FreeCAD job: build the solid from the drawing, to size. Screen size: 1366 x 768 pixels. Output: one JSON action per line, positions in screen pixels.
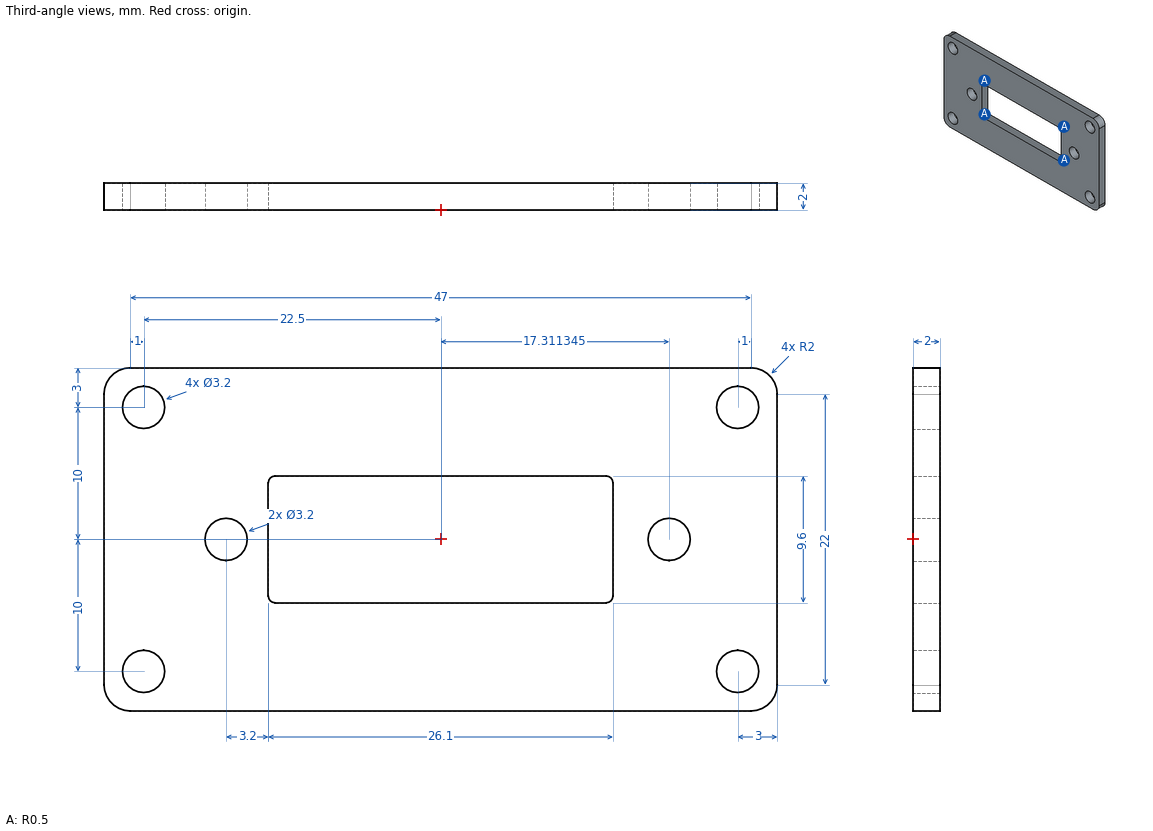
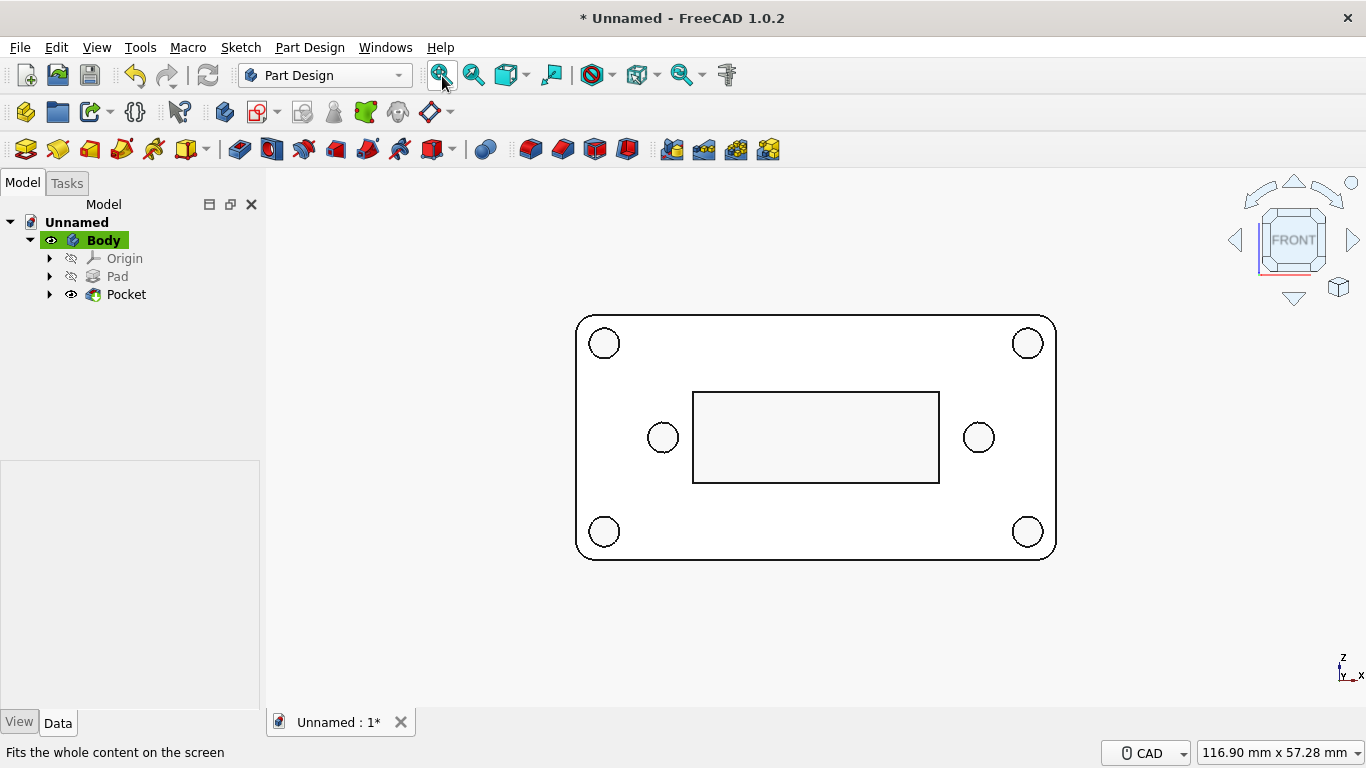
{"action": "key", "text": "3"}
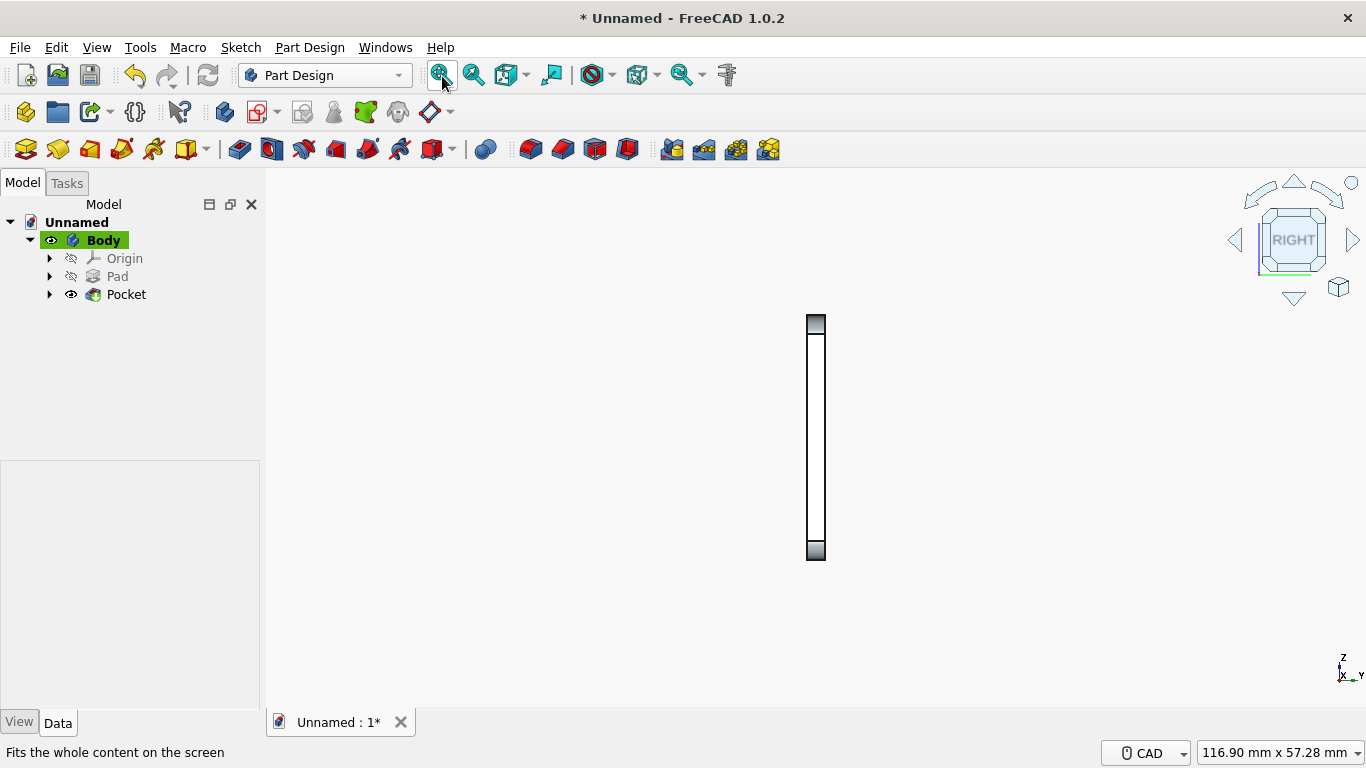
{"action": "scroll", "coordinate": [816, 391], "scroll_direction": "up", "scroll_amount": 4}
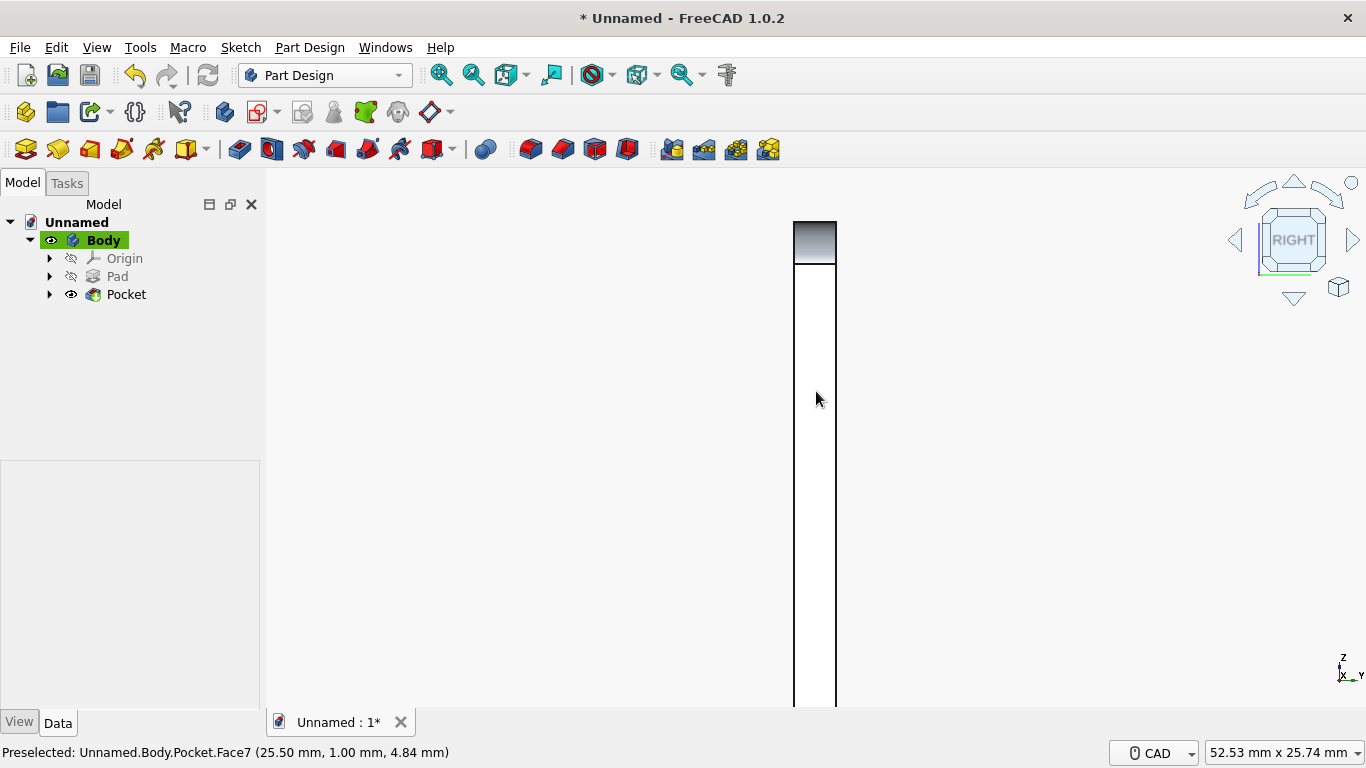
{"action": "left_click", "coordinate": [442, 76]}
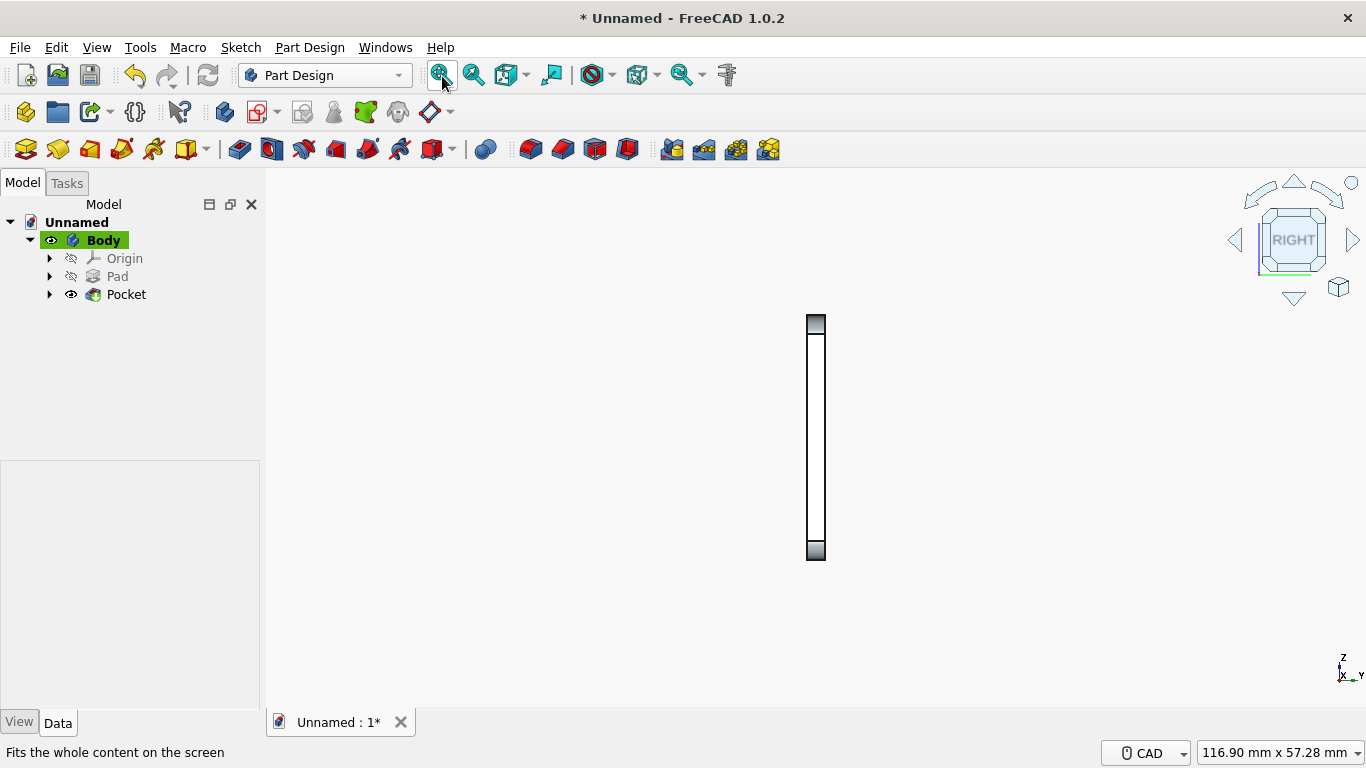
{"action": "key", "text": "5"}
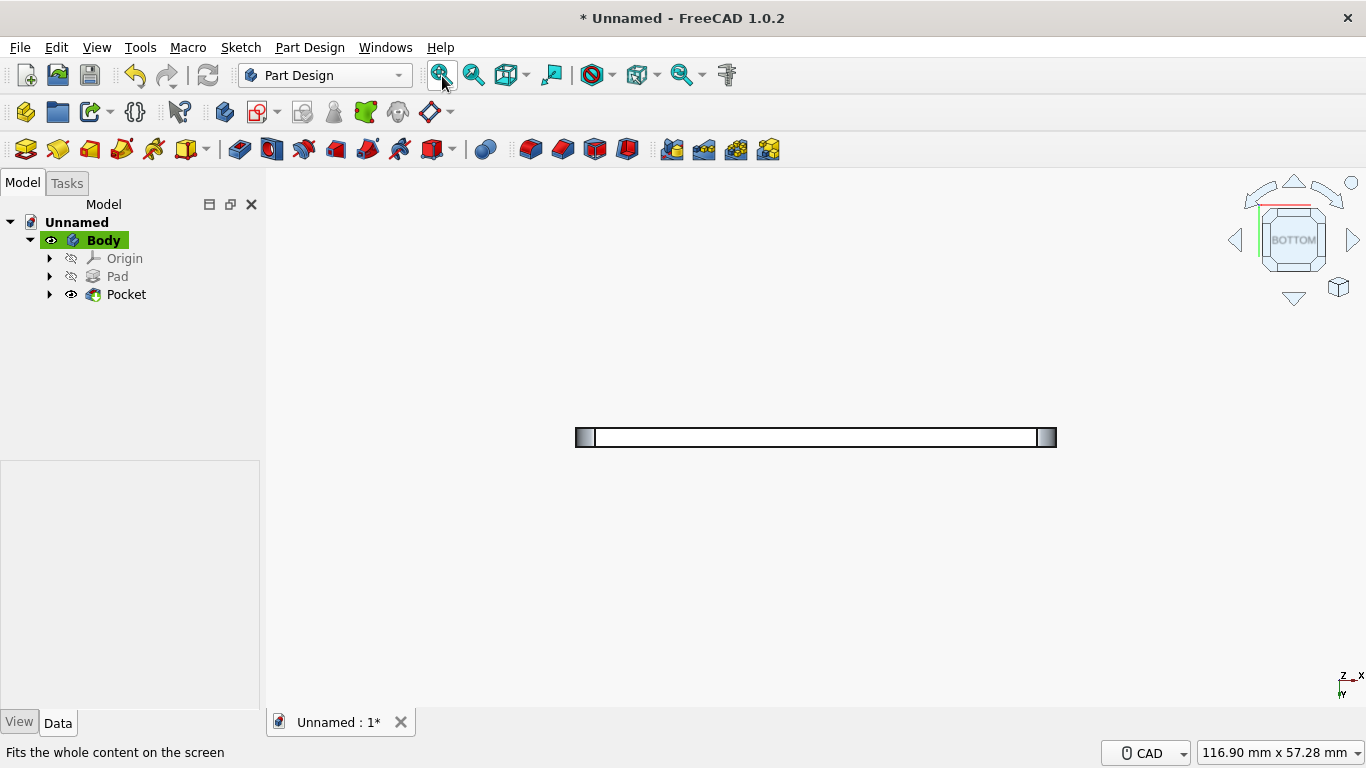
{"action": "left_click", "coordinate": [442, 76]}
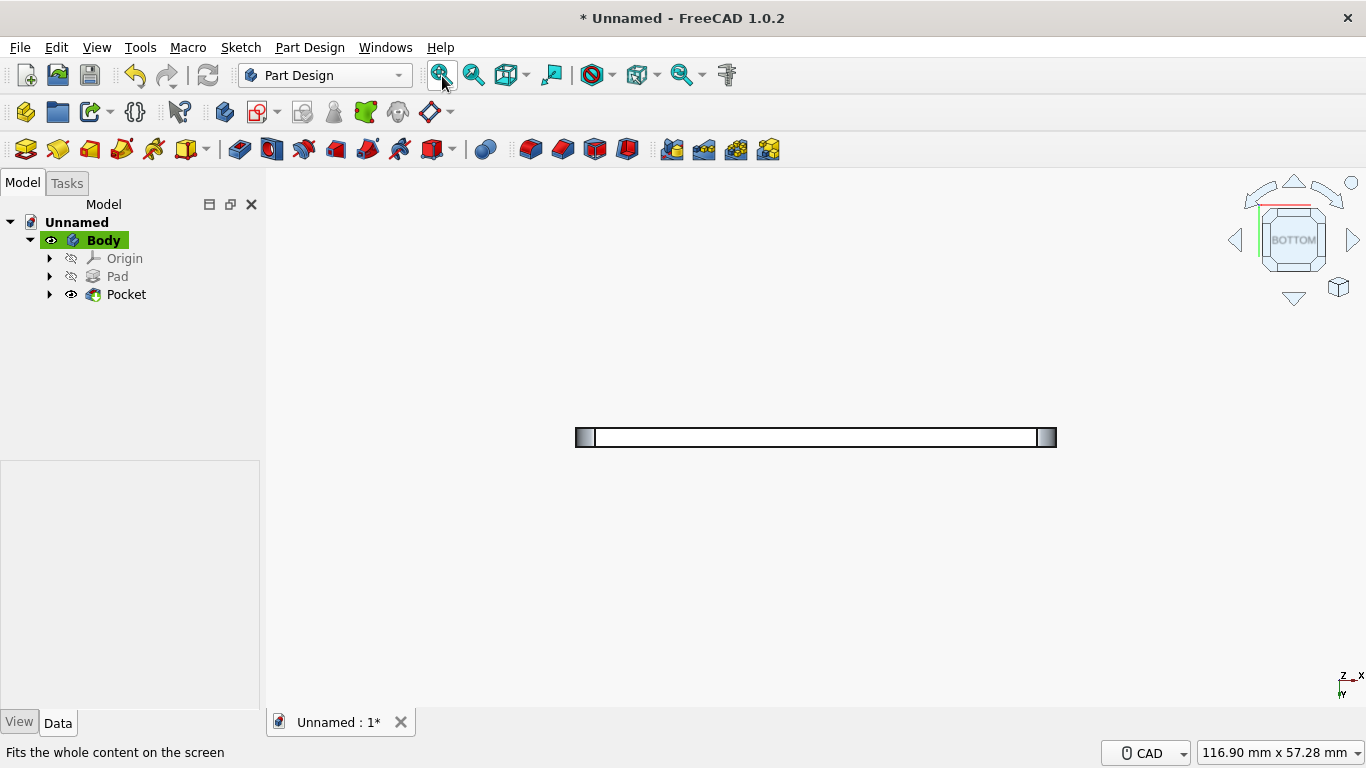
{"action": "scroll", "coordinate": [939, 436], "scroll_direction": "up", "scroll_amount": 4}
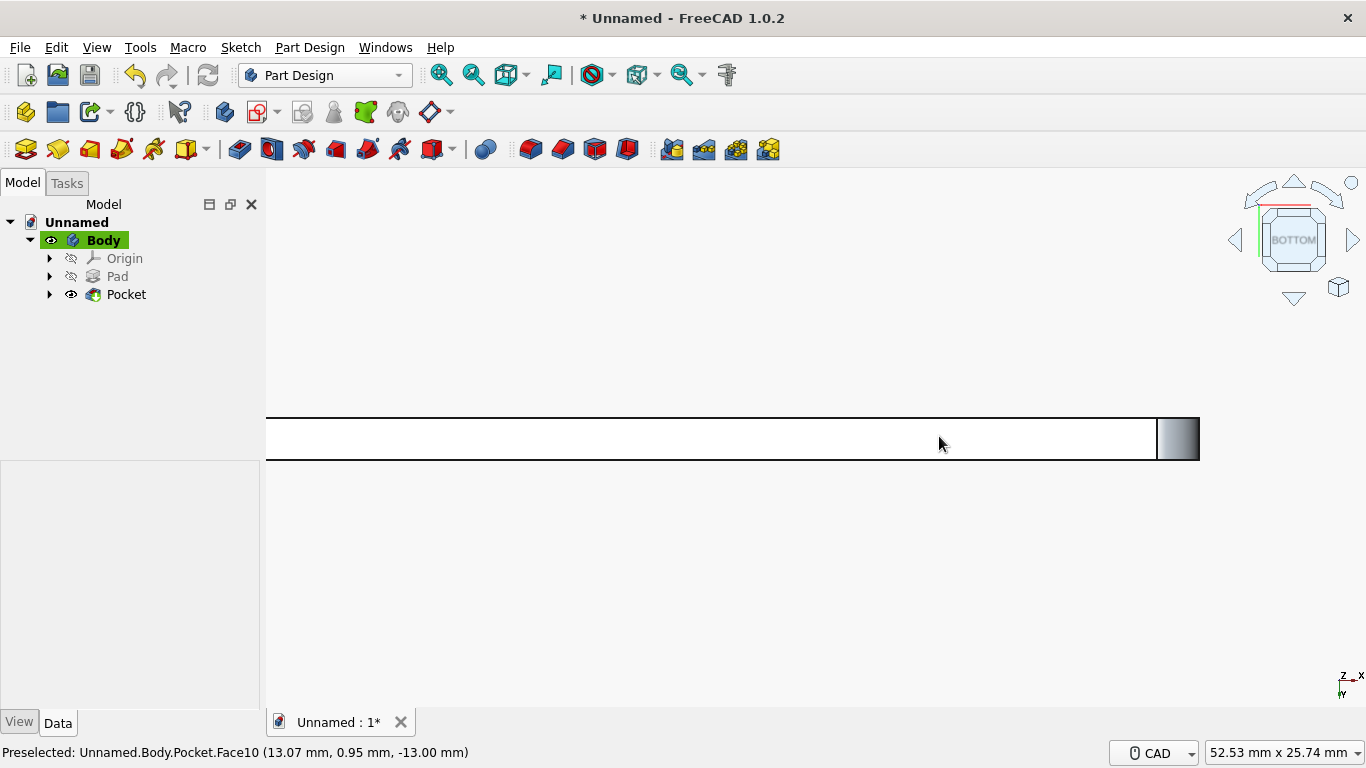
{"action": "left_click", "coordinate": [442, 76]}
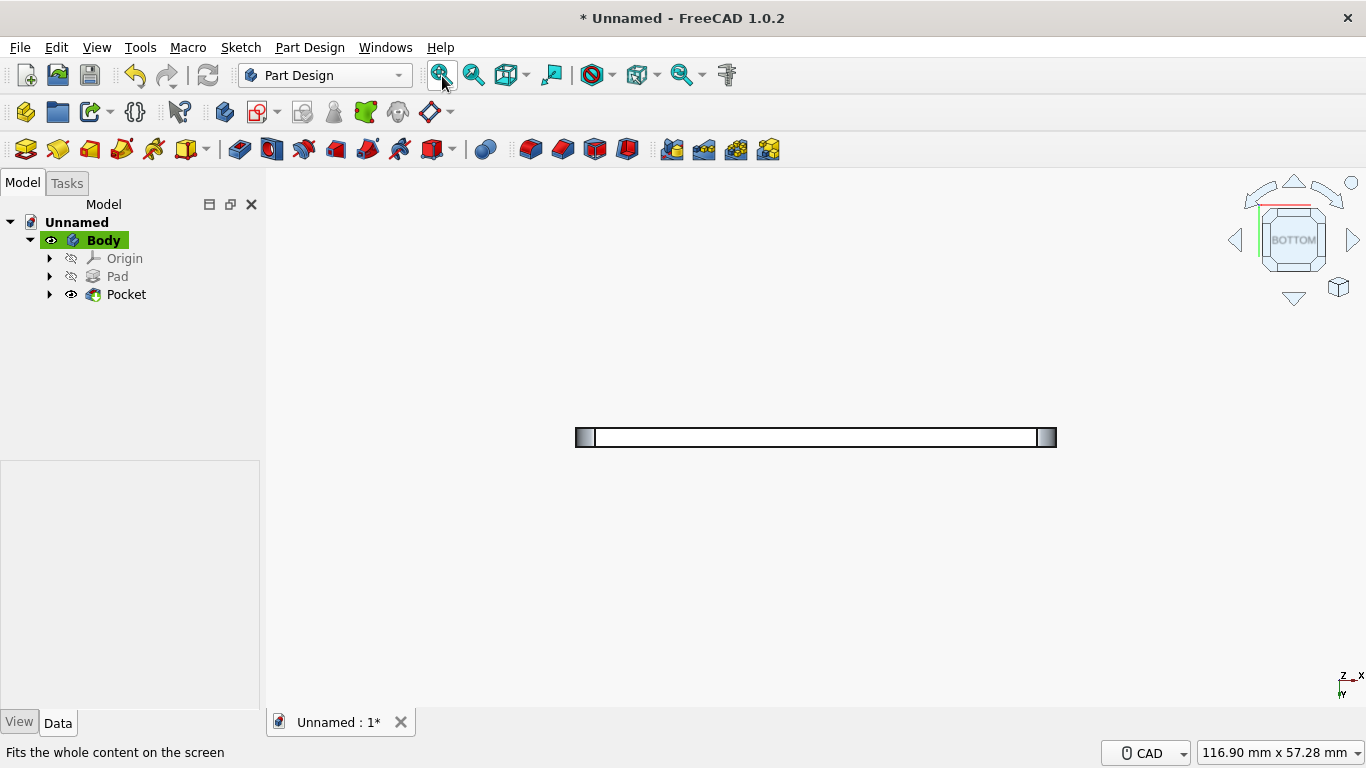
{"action": "key", "text": "4"}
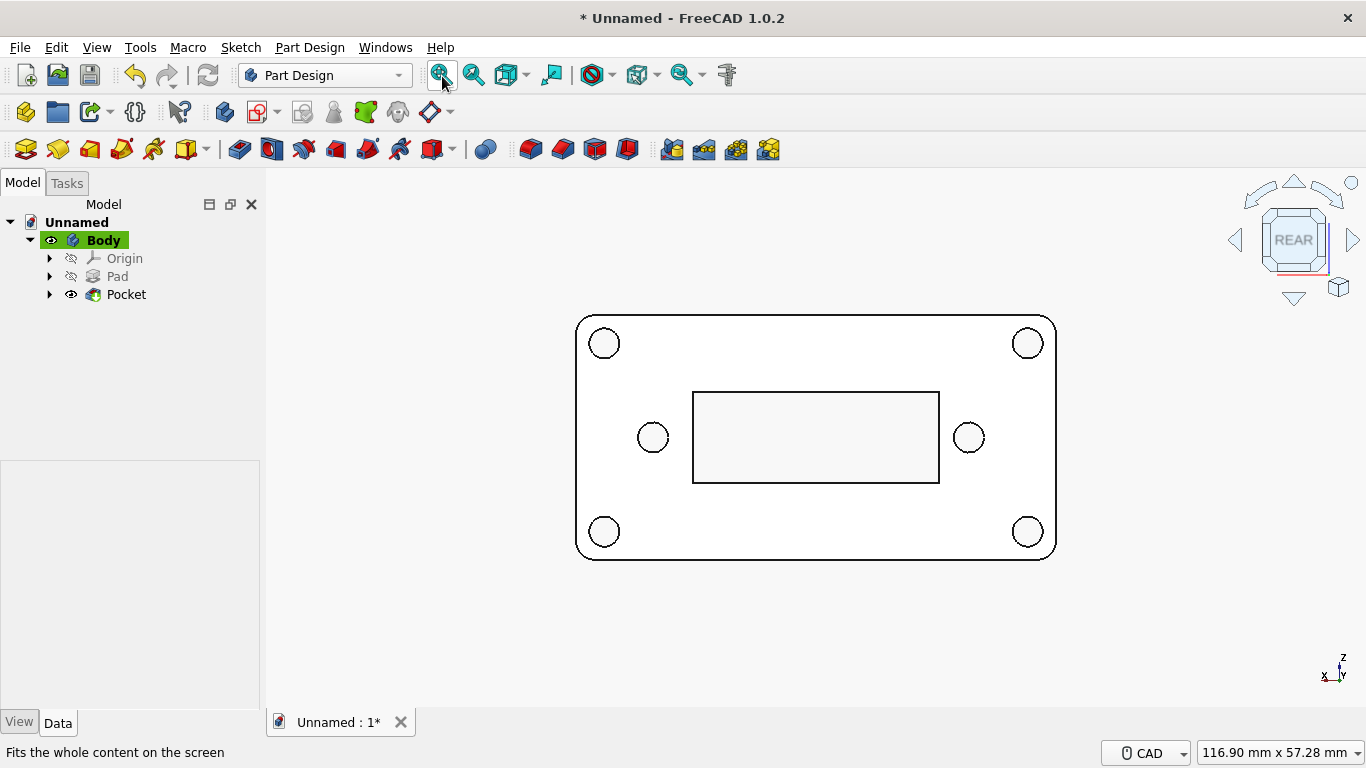
{"action": "scroll", "coordinate": [693, 391], "scroll_direction": "up", "scroll_amount": 4}